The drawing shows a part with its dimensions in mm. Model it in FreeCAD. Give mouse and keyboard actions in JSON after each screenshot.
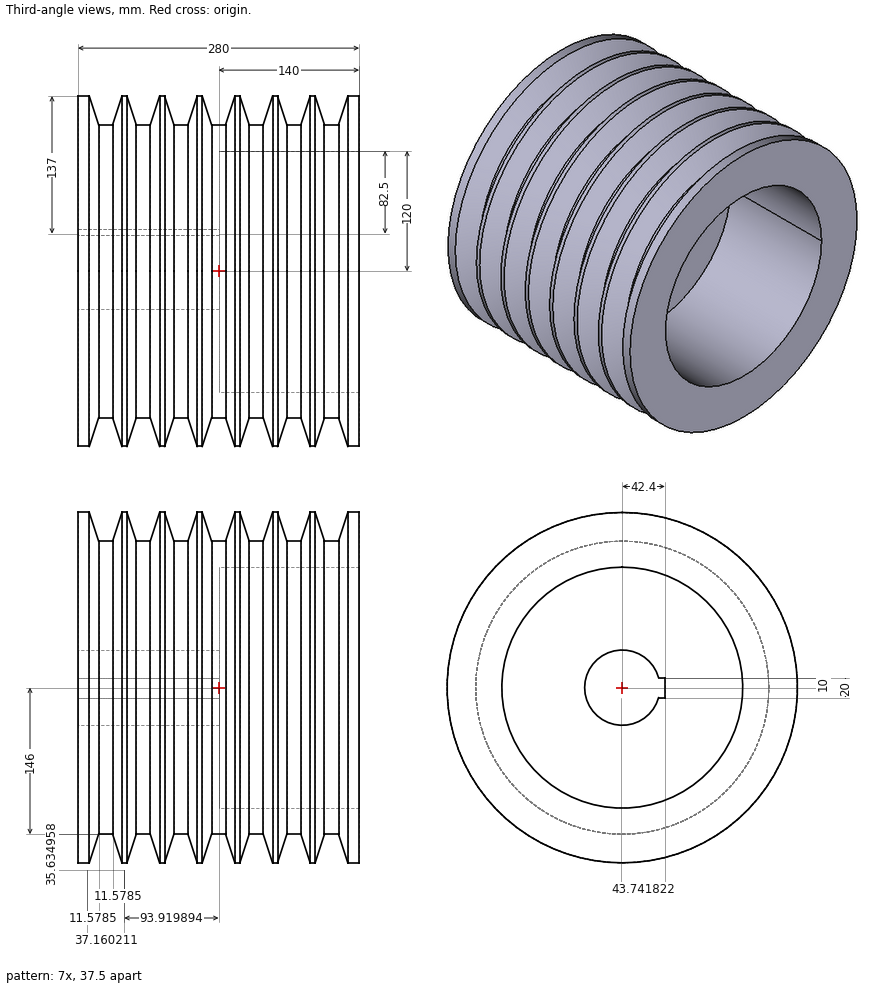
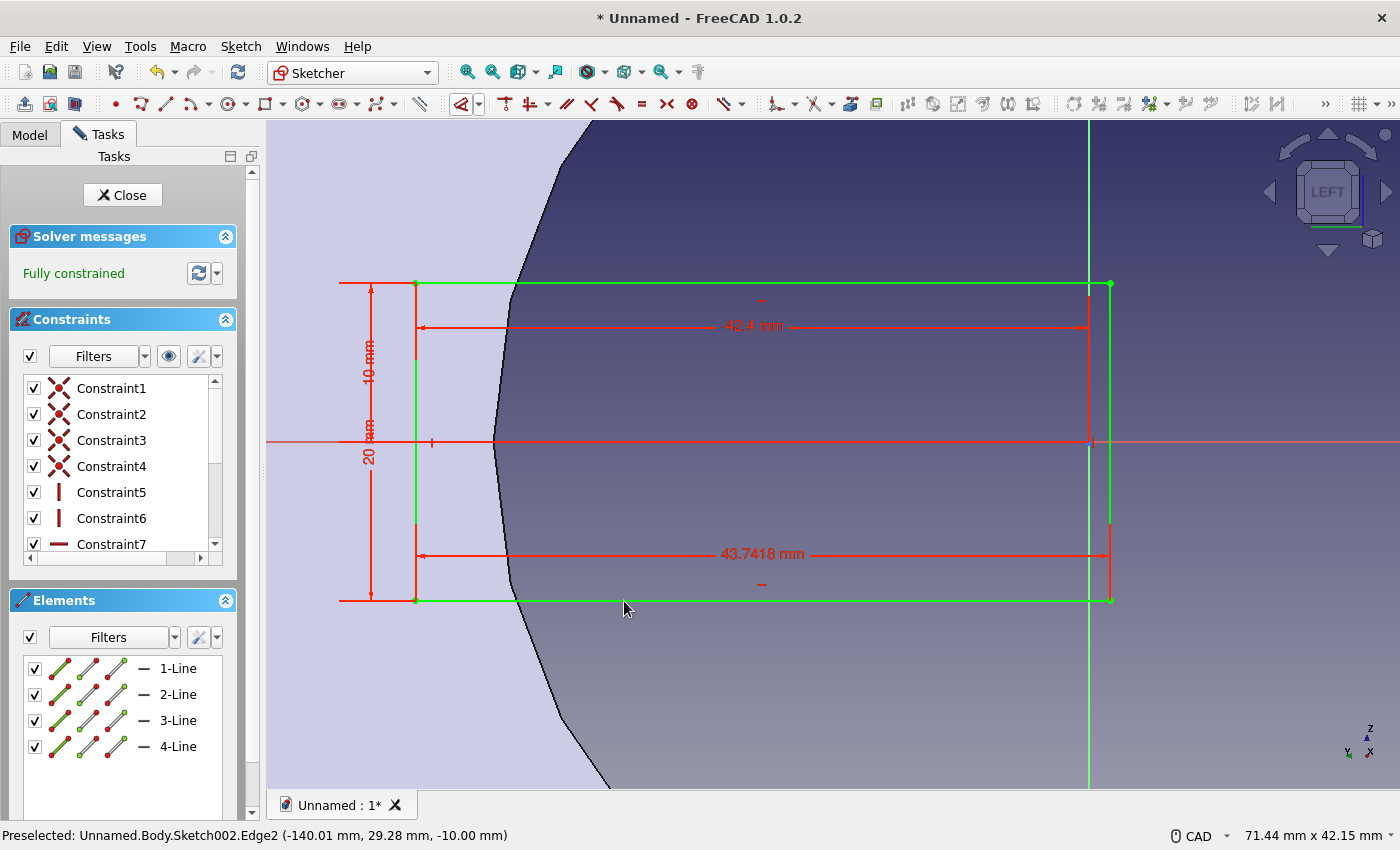
{"action": "left_click", "coordinate": [123, 195]}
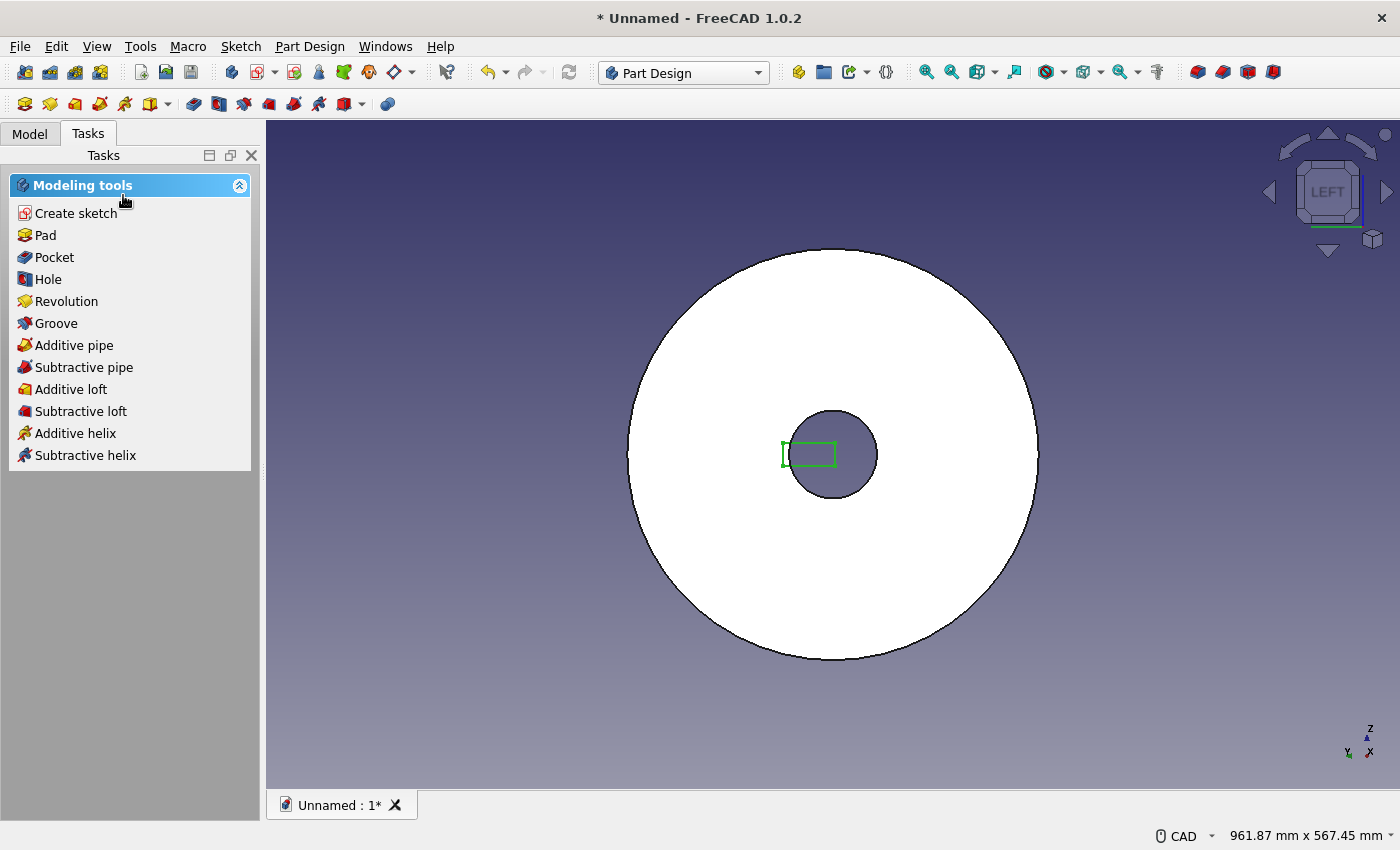
{"action": "left_click", "coordinate": [194, 104]}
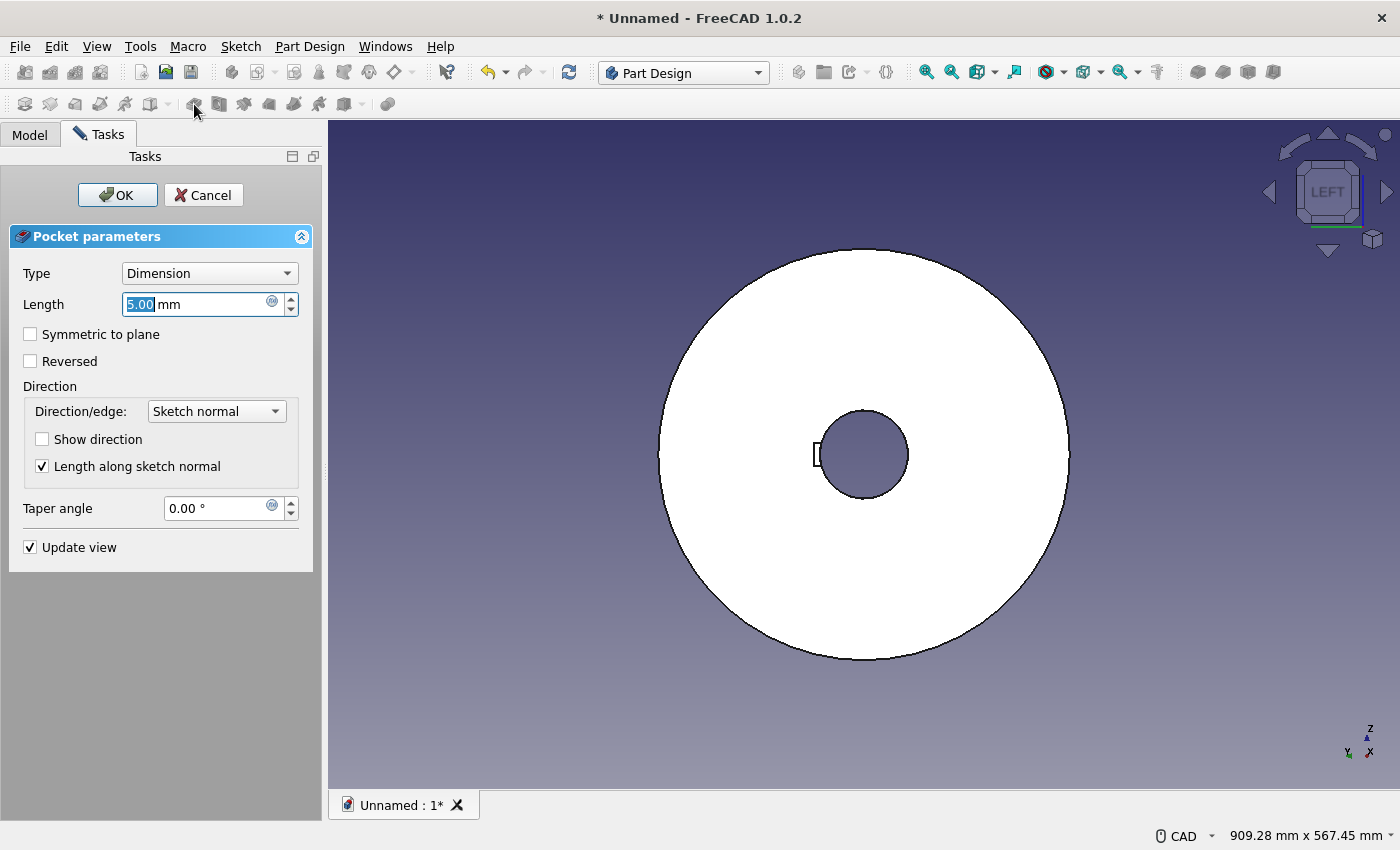
{"action": "left_click", "coordinate": [210, 274]}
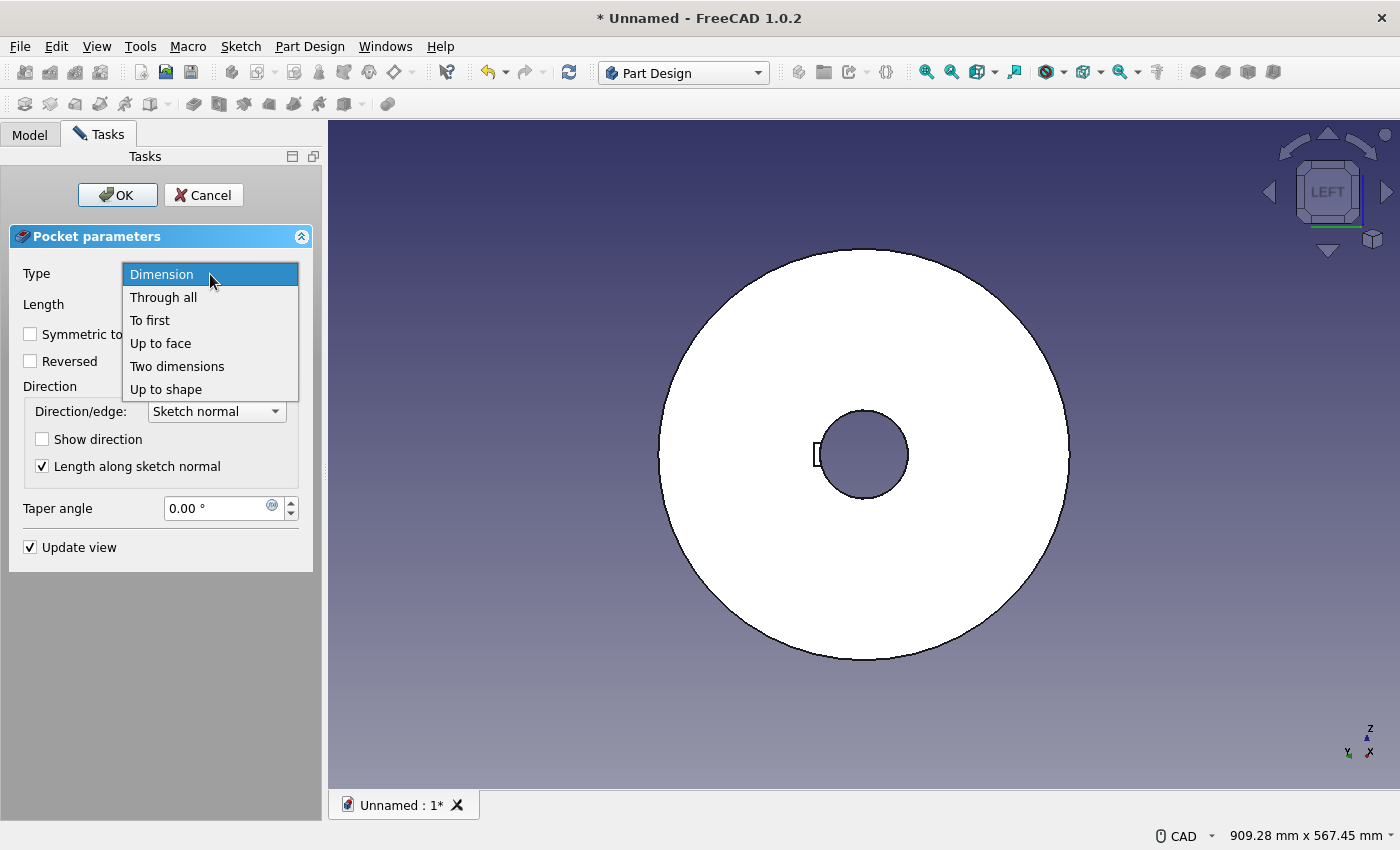
{"action": "left_click", "coordinate": [208, 298]}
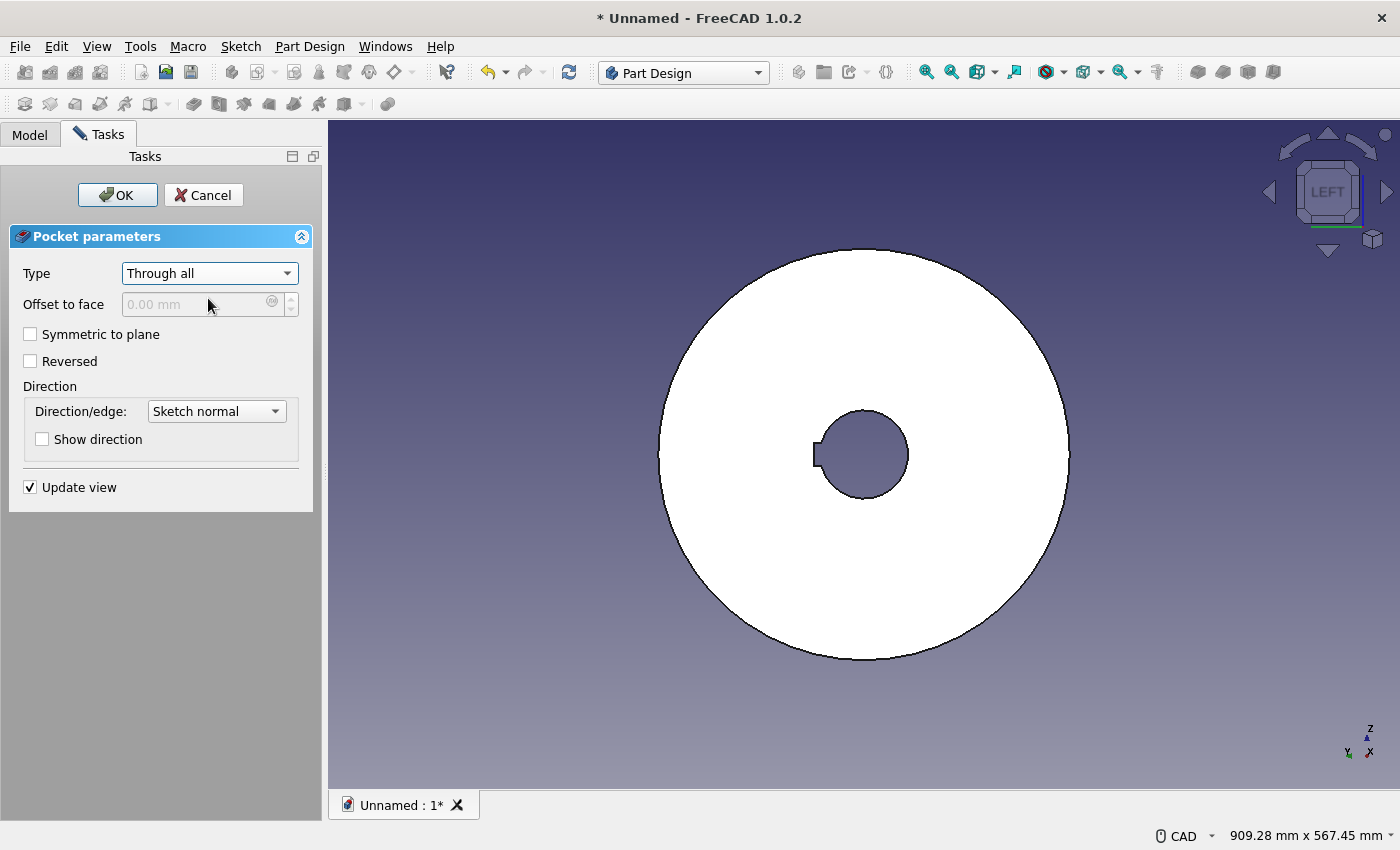
{"action": "left_click", "coordinate": [118, 195]}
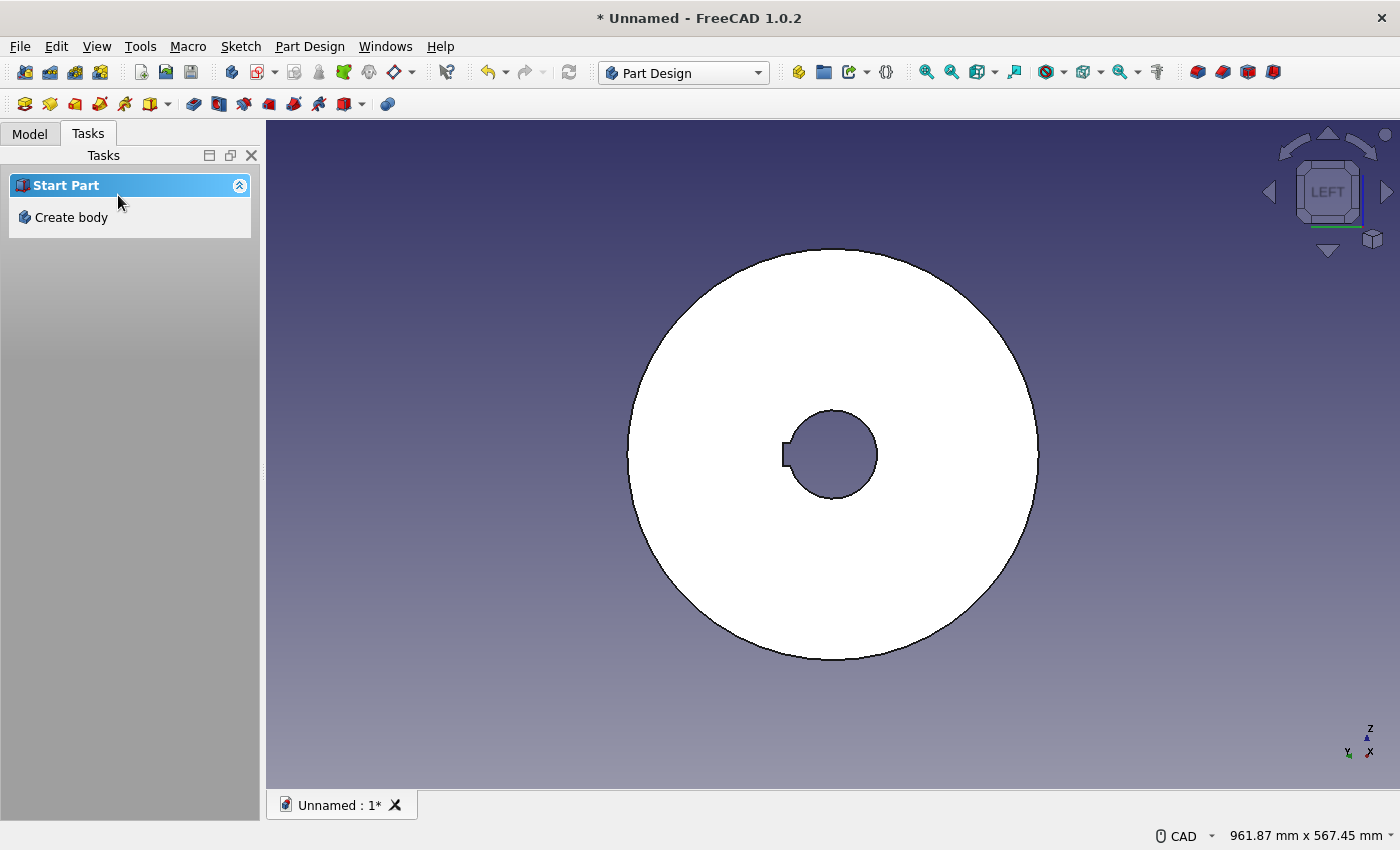
{"action": "left_click", "coordinate": [30, 134]}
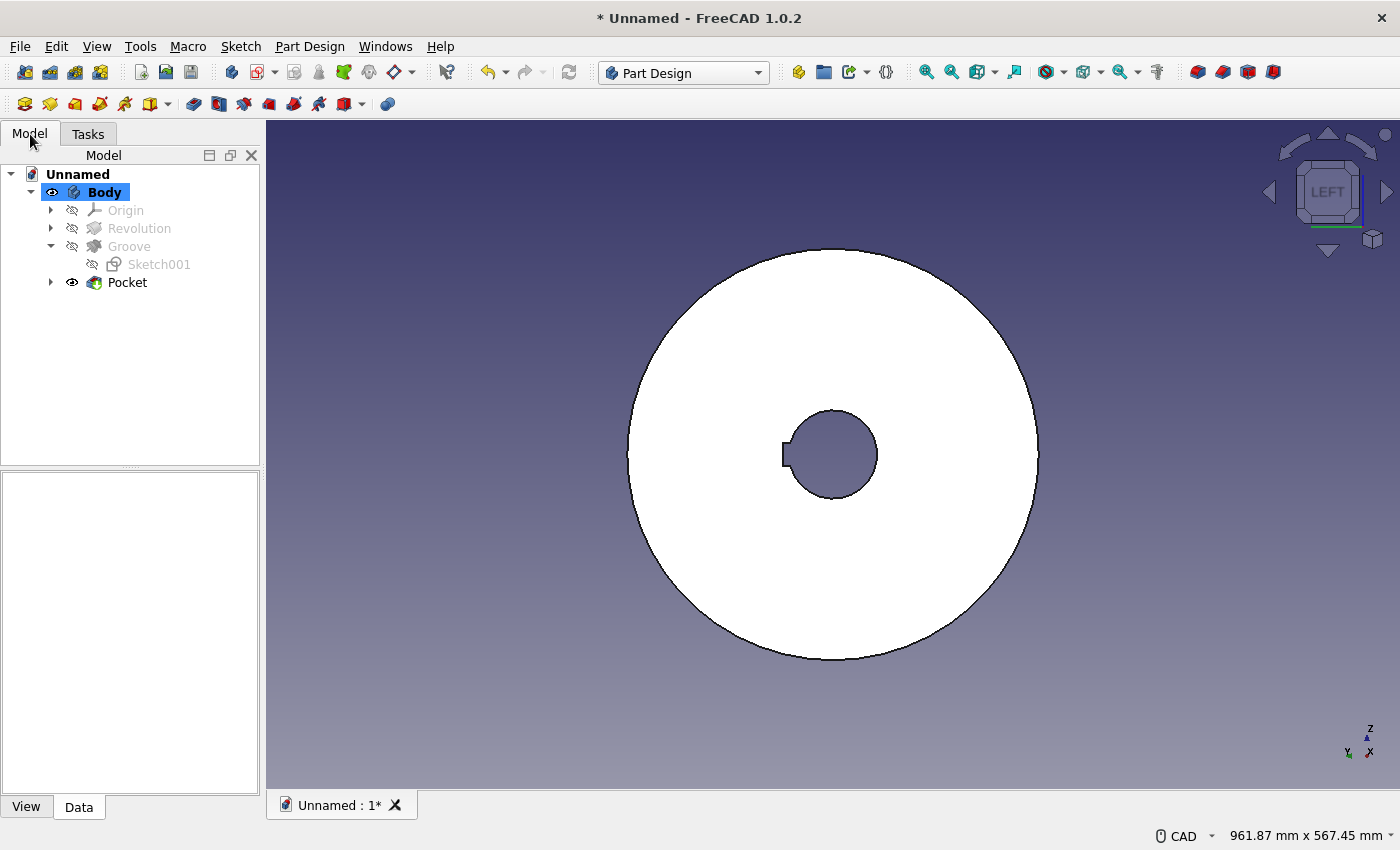
{"action": "left_click", "coordinate": [117, 246]}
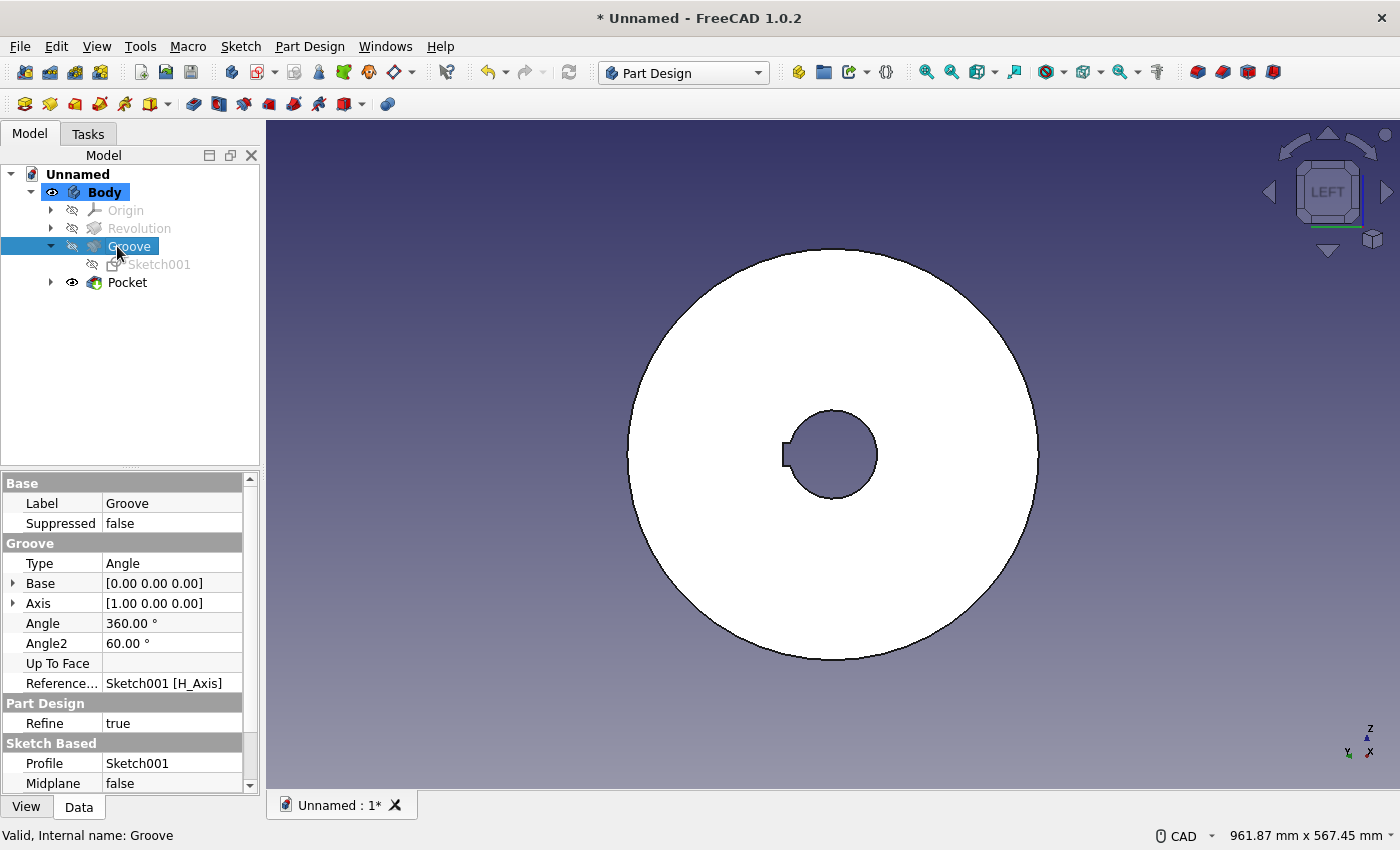
{"action": "left_click", "coordinate": [50, 72]}